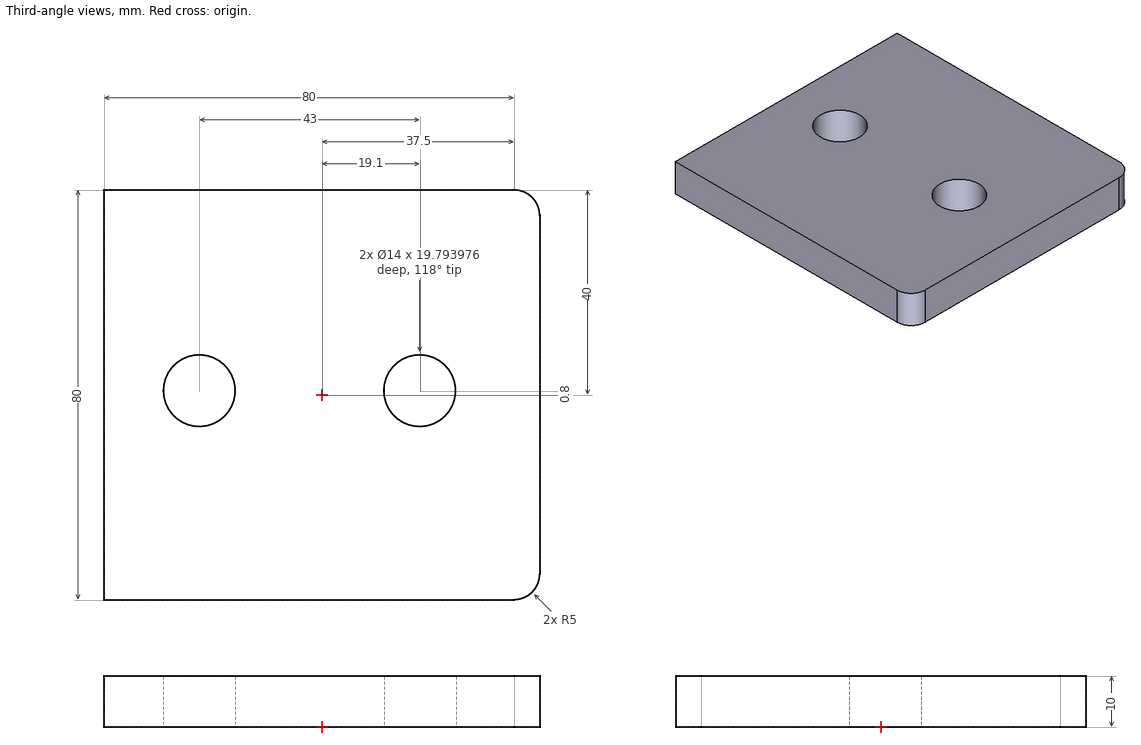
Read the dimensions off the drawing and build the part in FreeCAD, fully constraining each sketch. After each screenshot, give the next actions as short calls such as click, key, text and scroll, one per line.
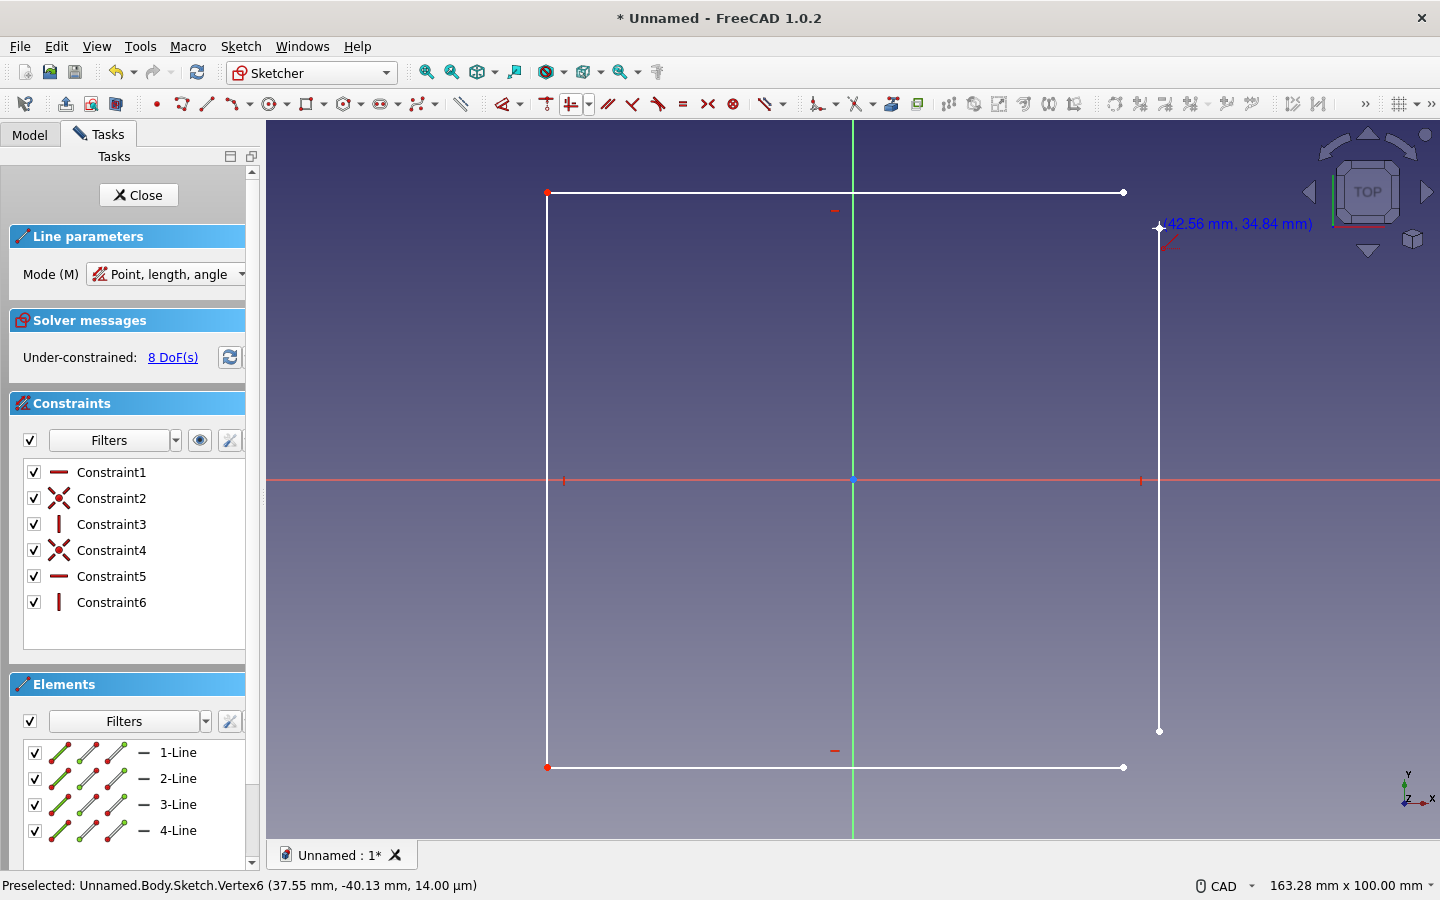
click(232, 104)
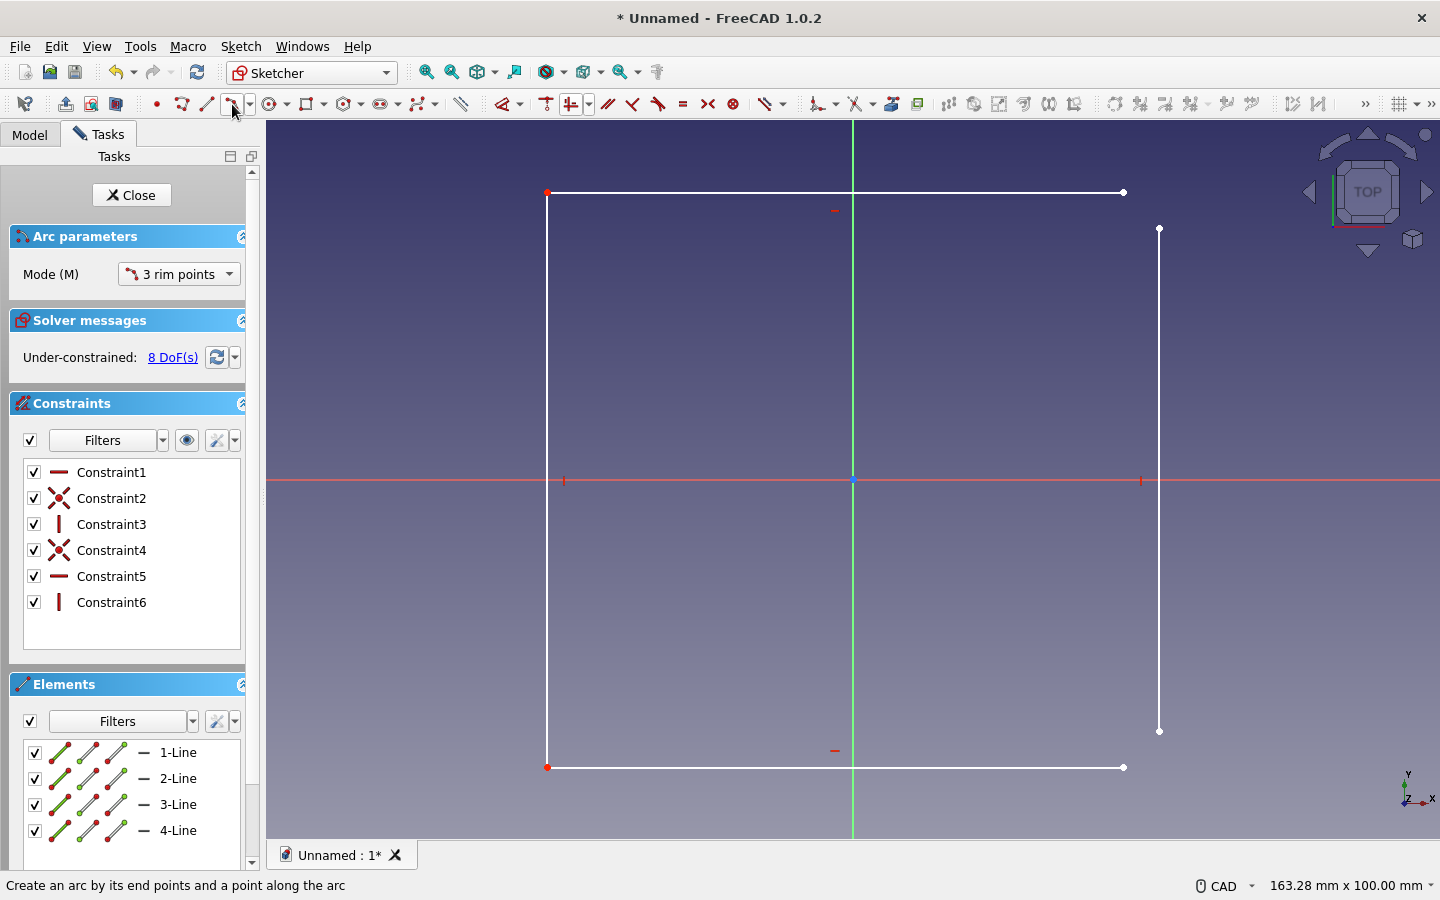
click(1123, 768)
click(1159, 732)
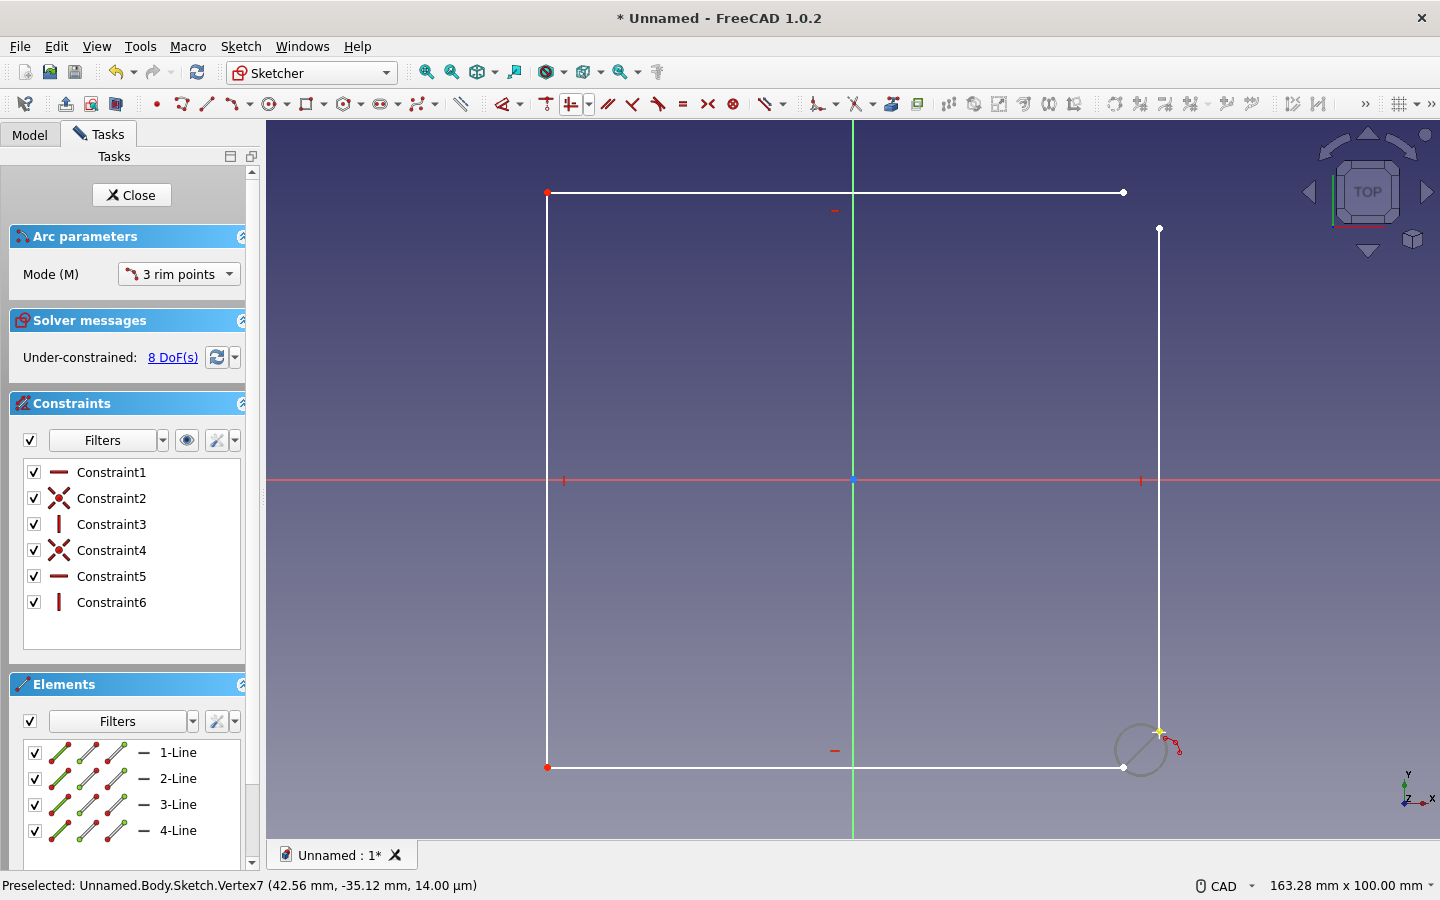
scroll(1148, 757, up, 3)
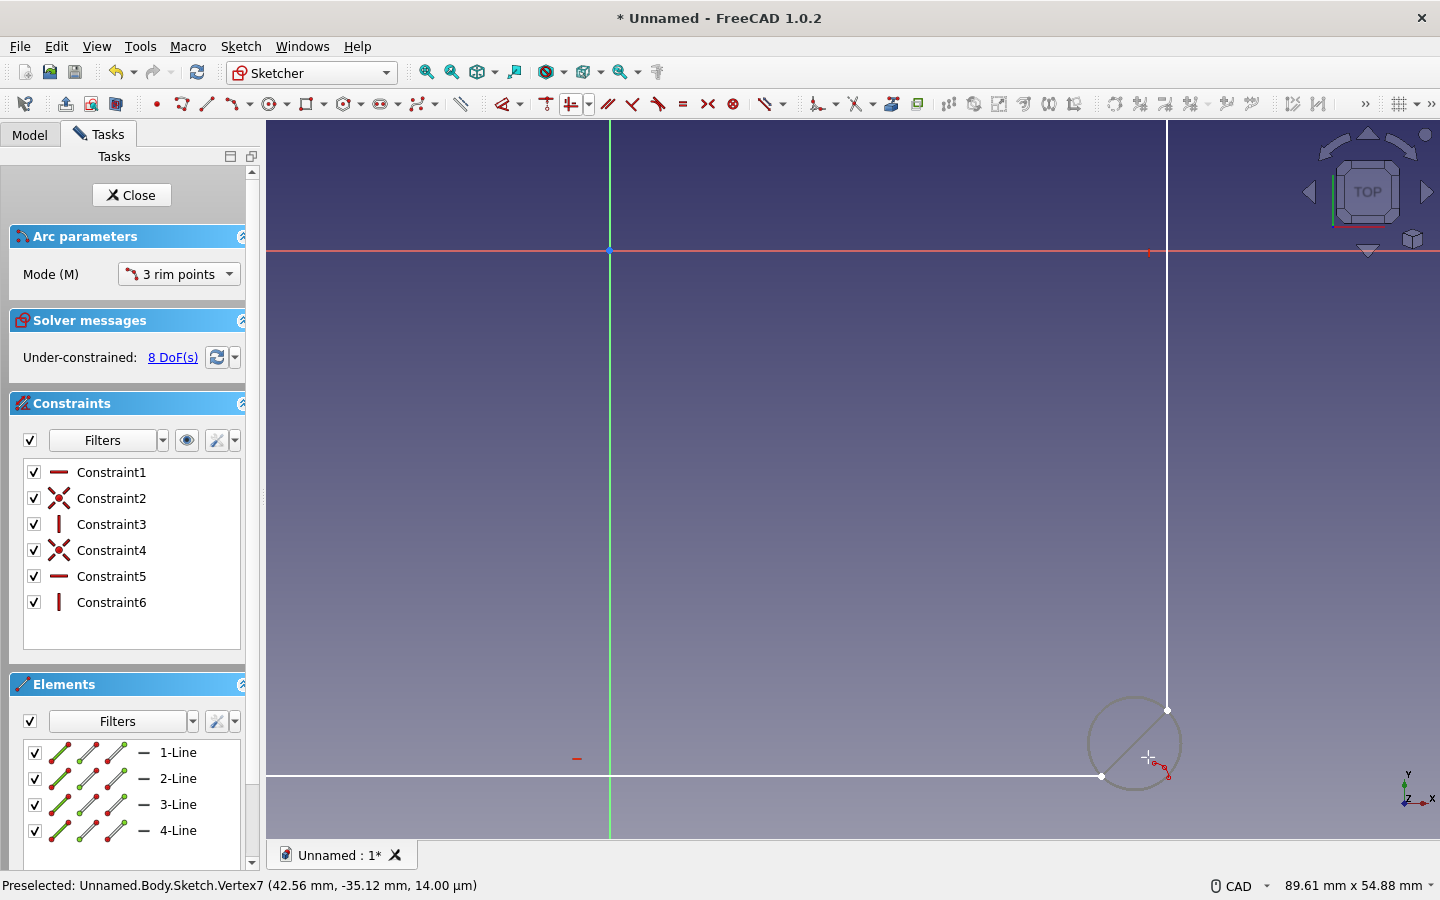
click(1147, 755)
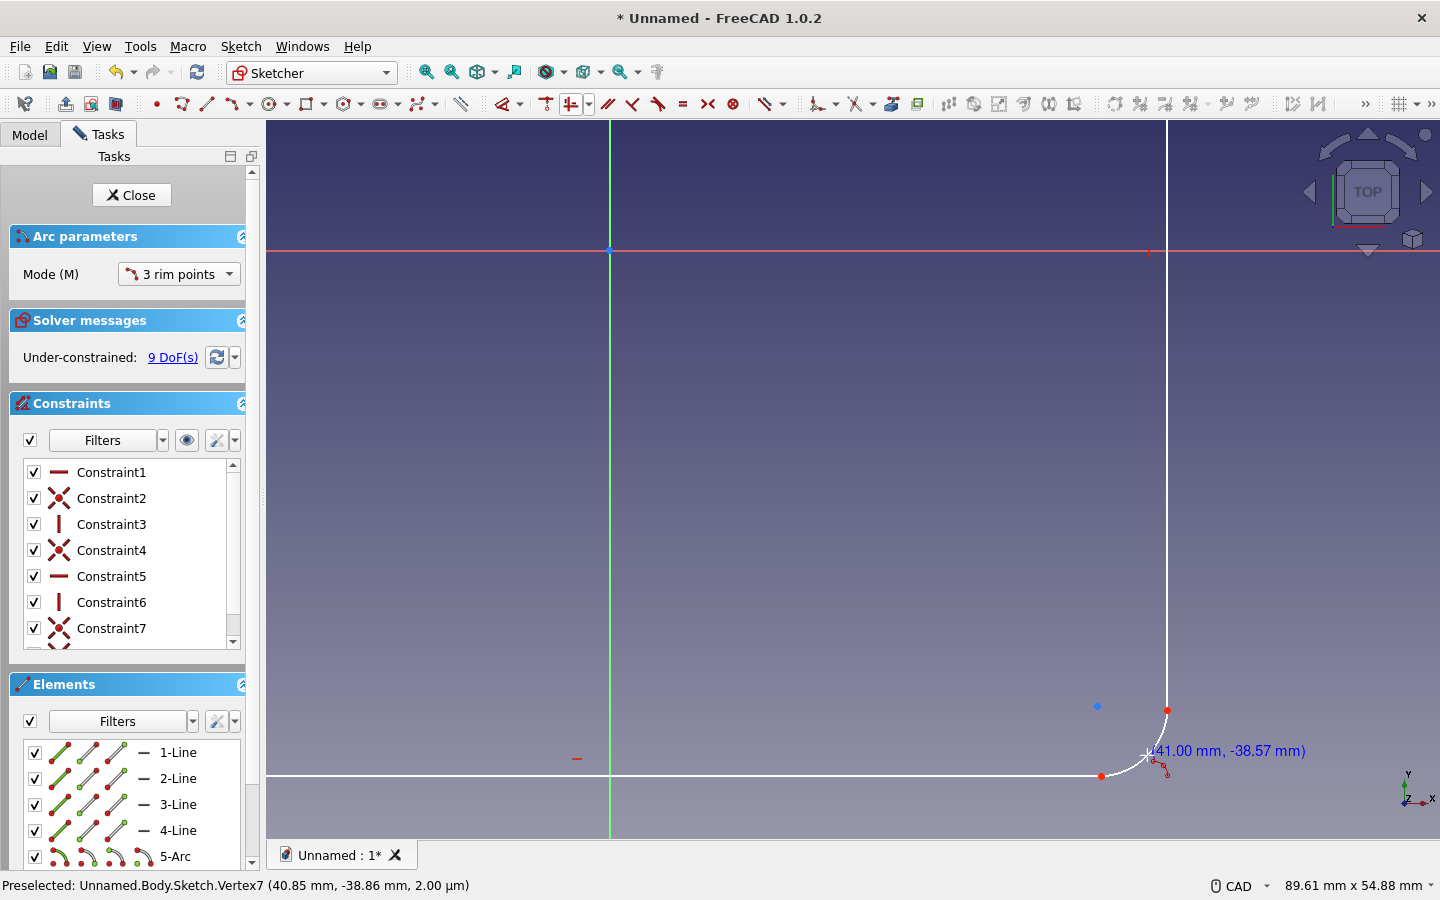
scroll(927, 666, down, 4)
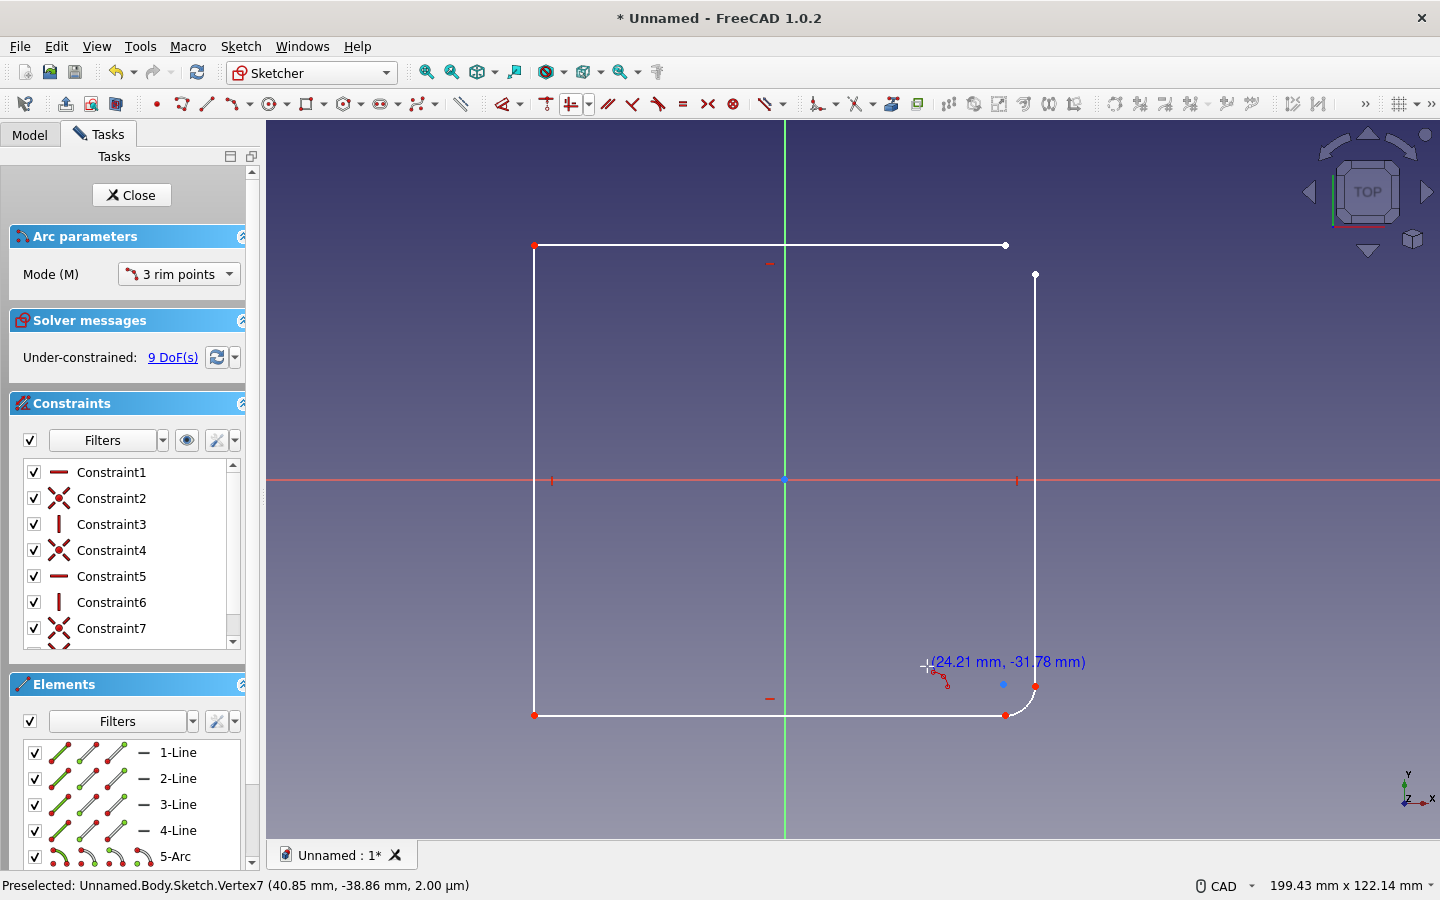
click(1035, 275)
click(1006, 245)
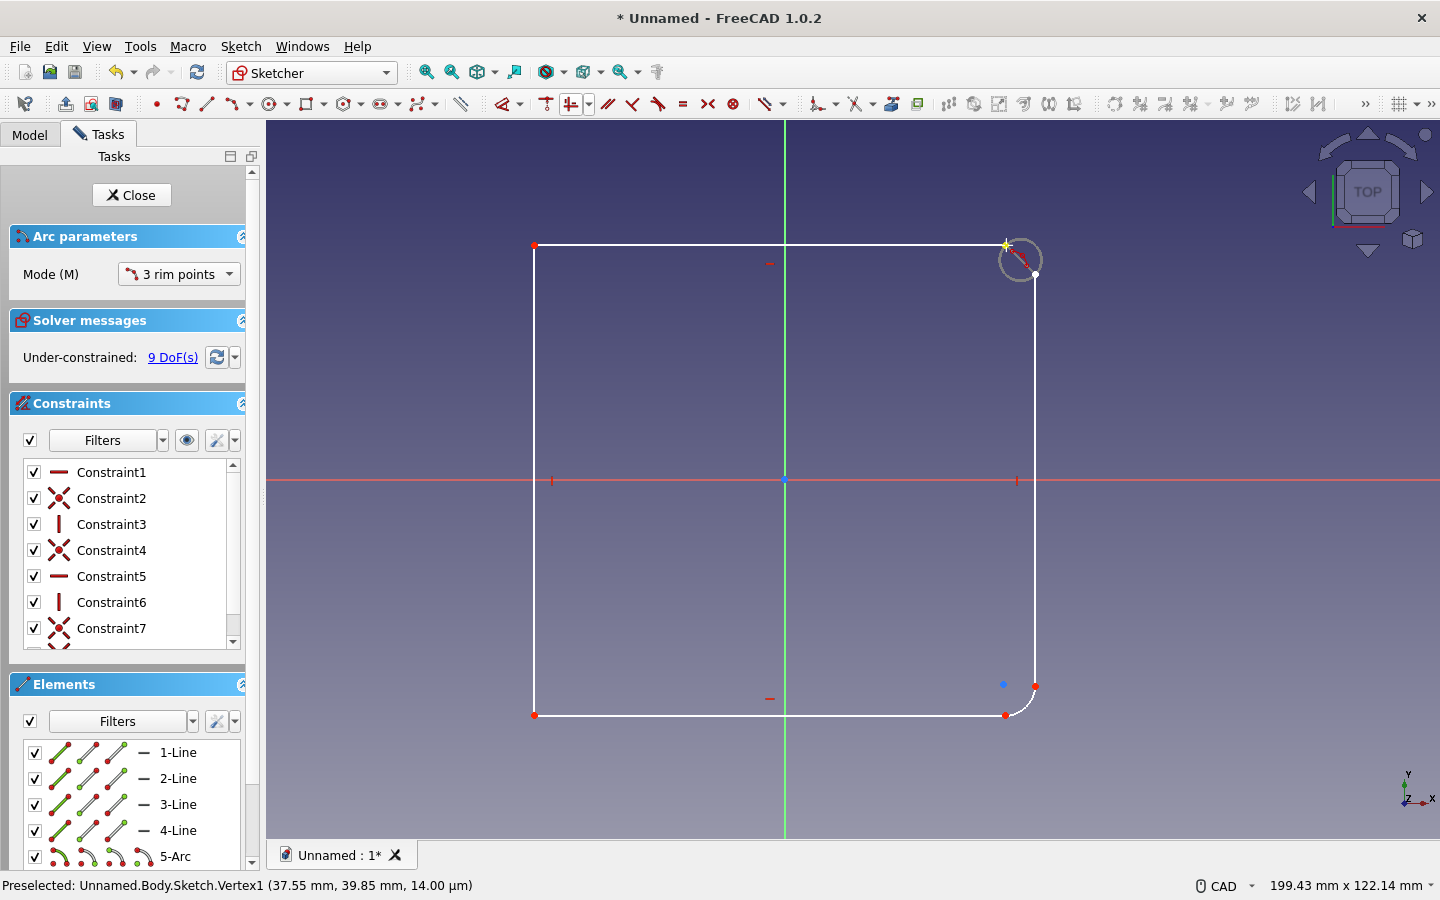
scroll(1026, 253, up, 4)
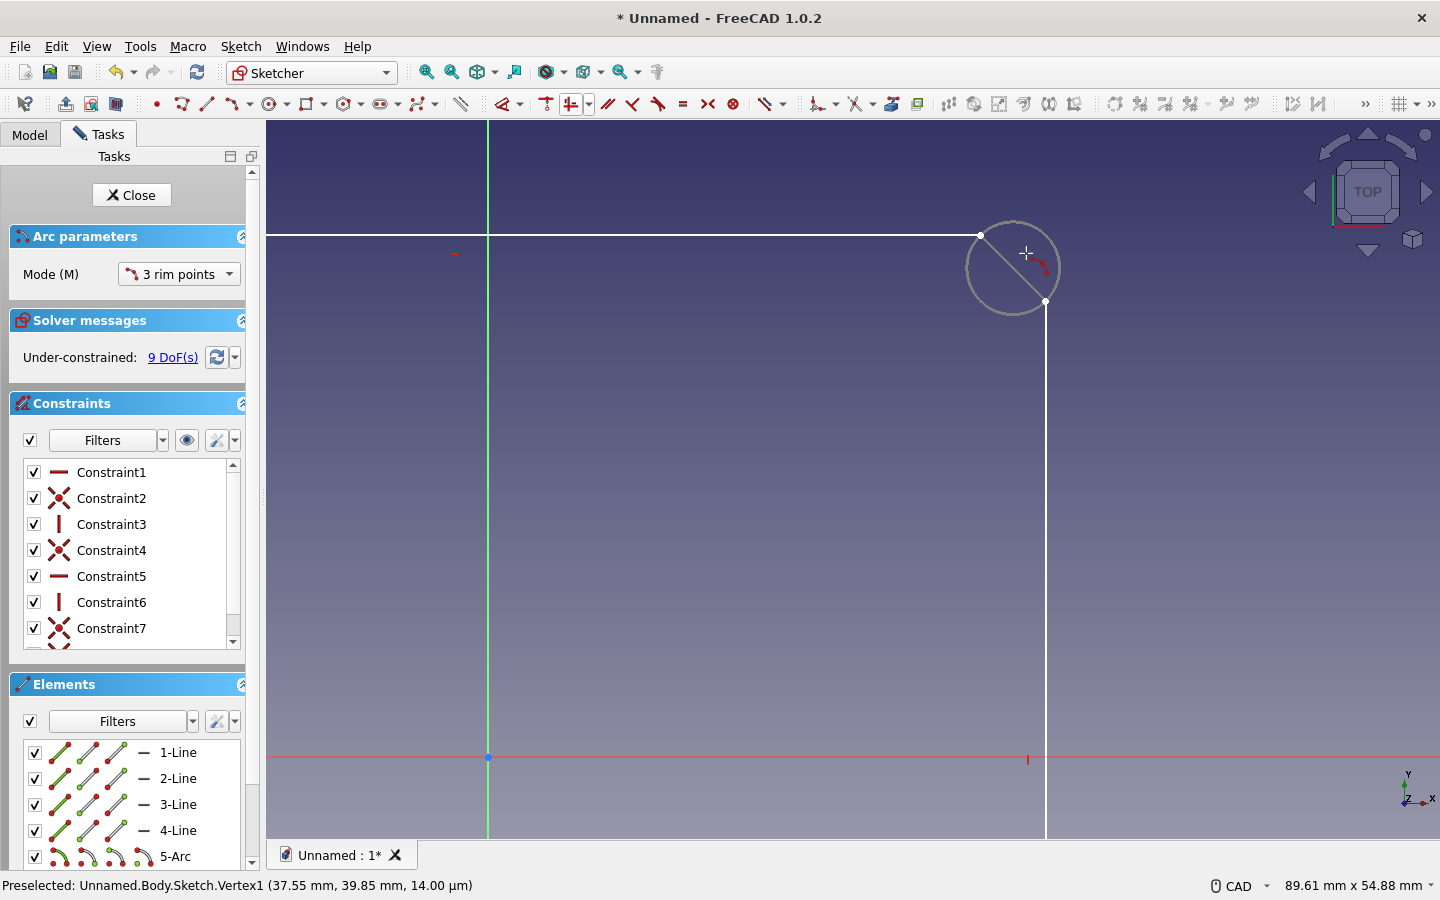
click(1026, 253)
key(Escape)